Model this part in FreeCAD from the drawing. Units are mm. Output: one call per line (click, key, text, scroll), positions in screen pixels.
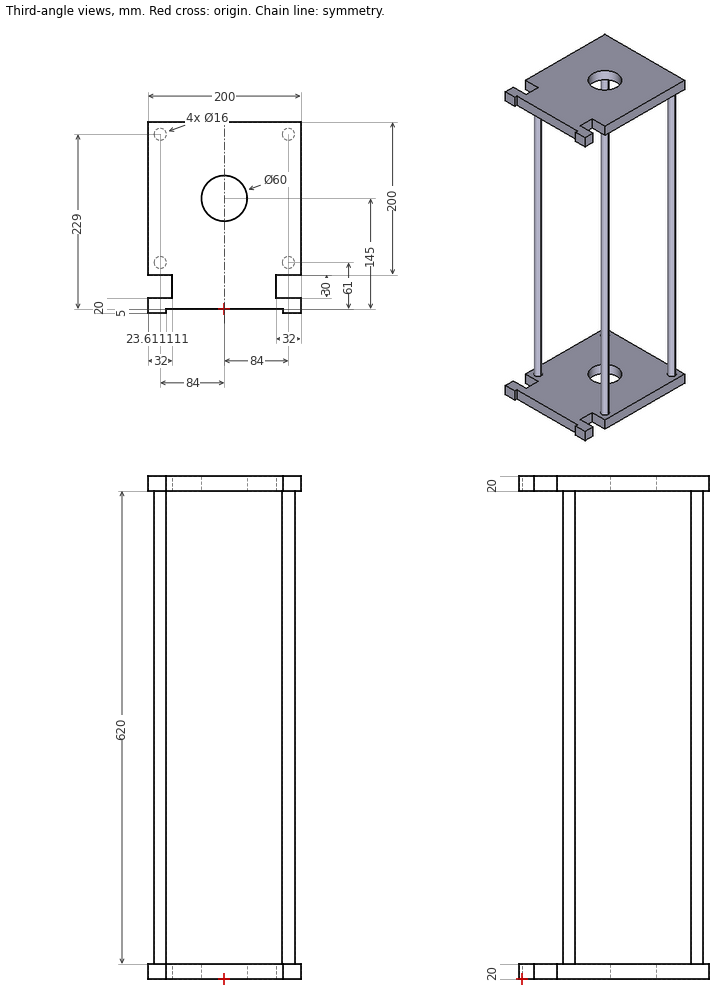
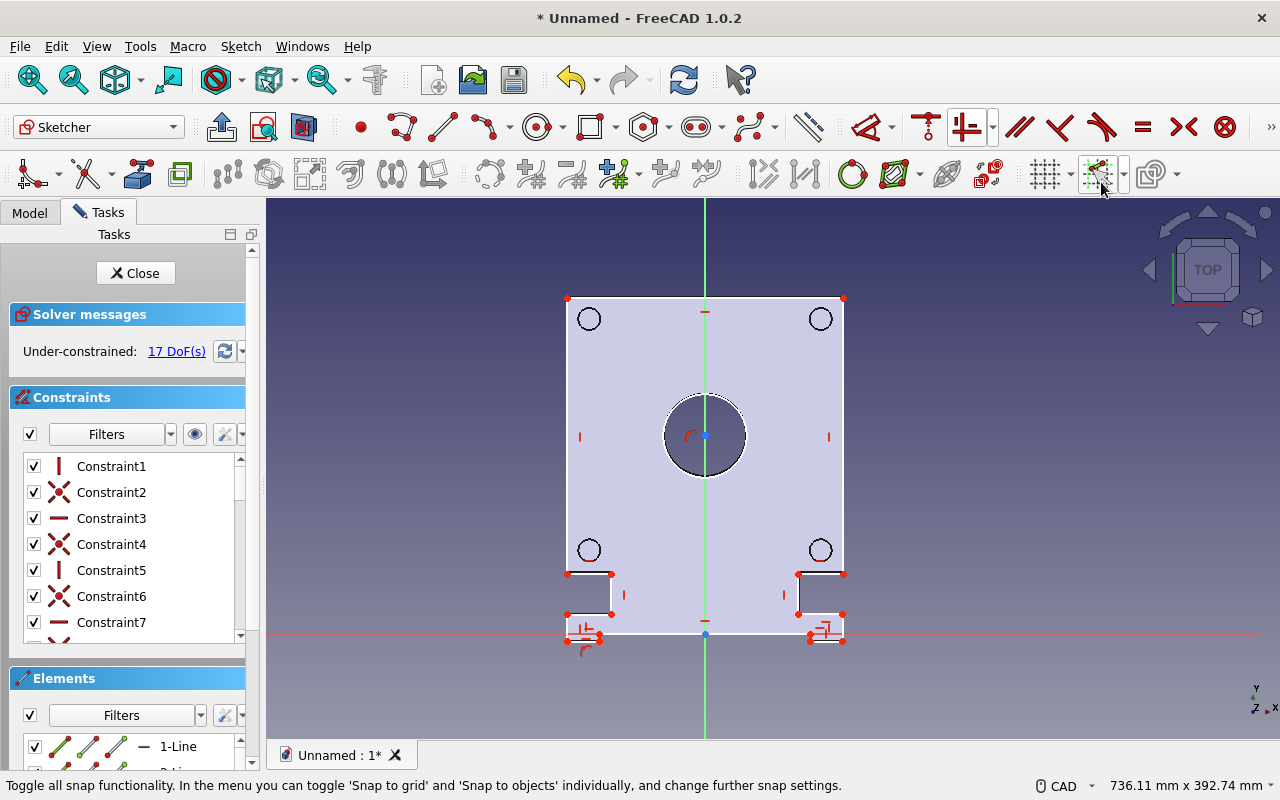
click(843, 574)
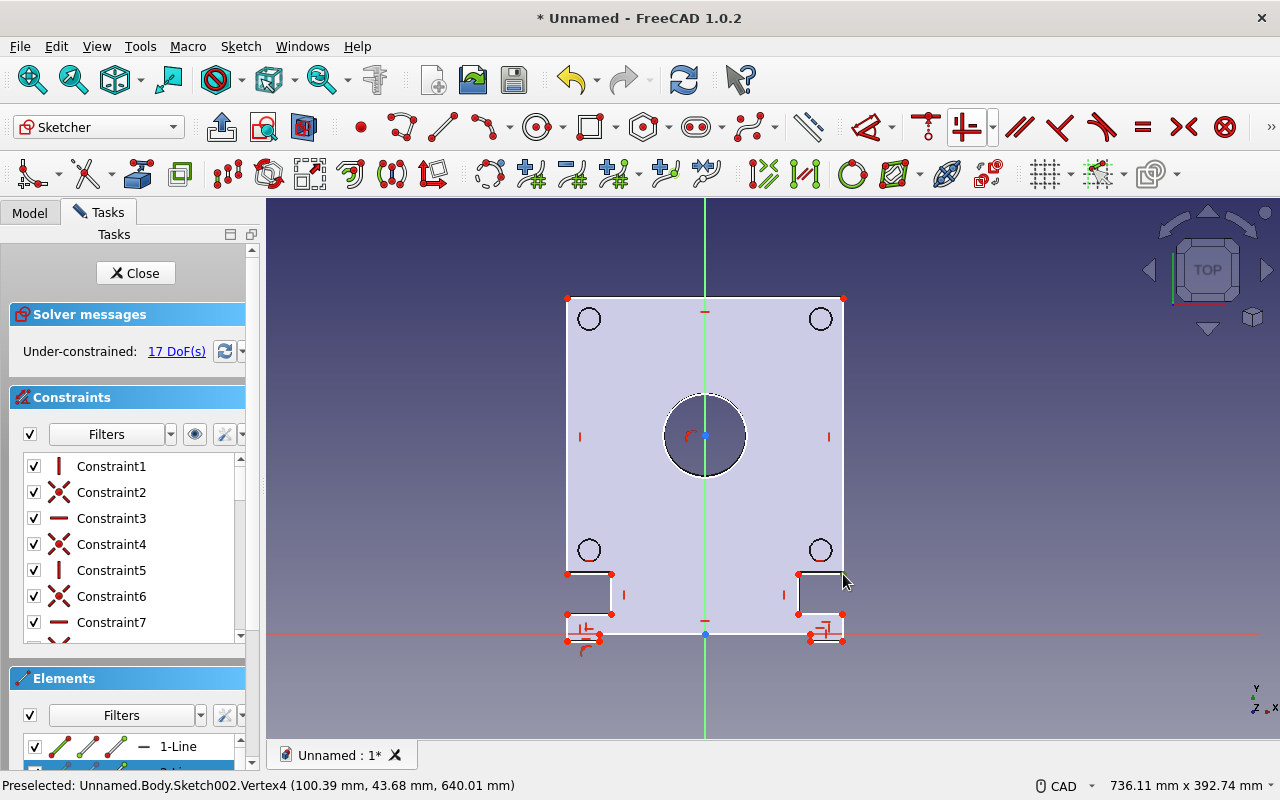
click(567, 574)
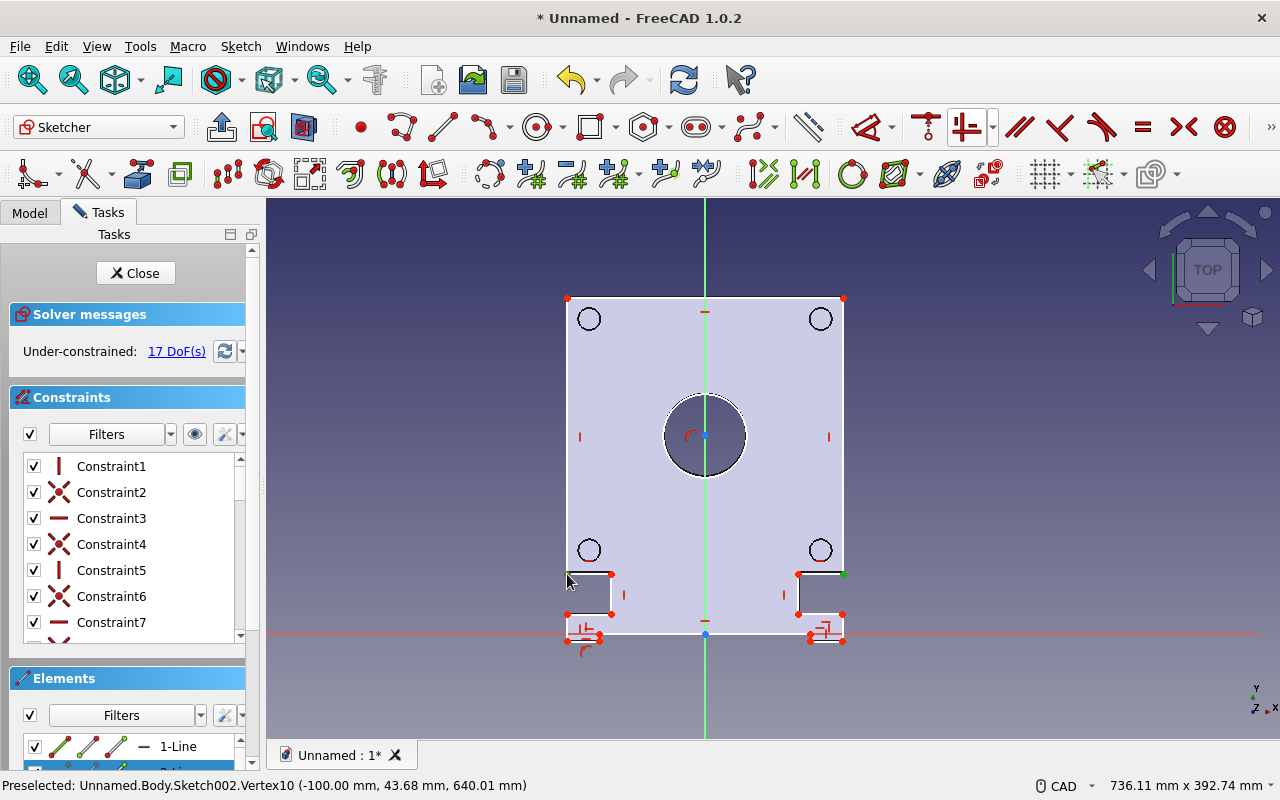
click(705, 676)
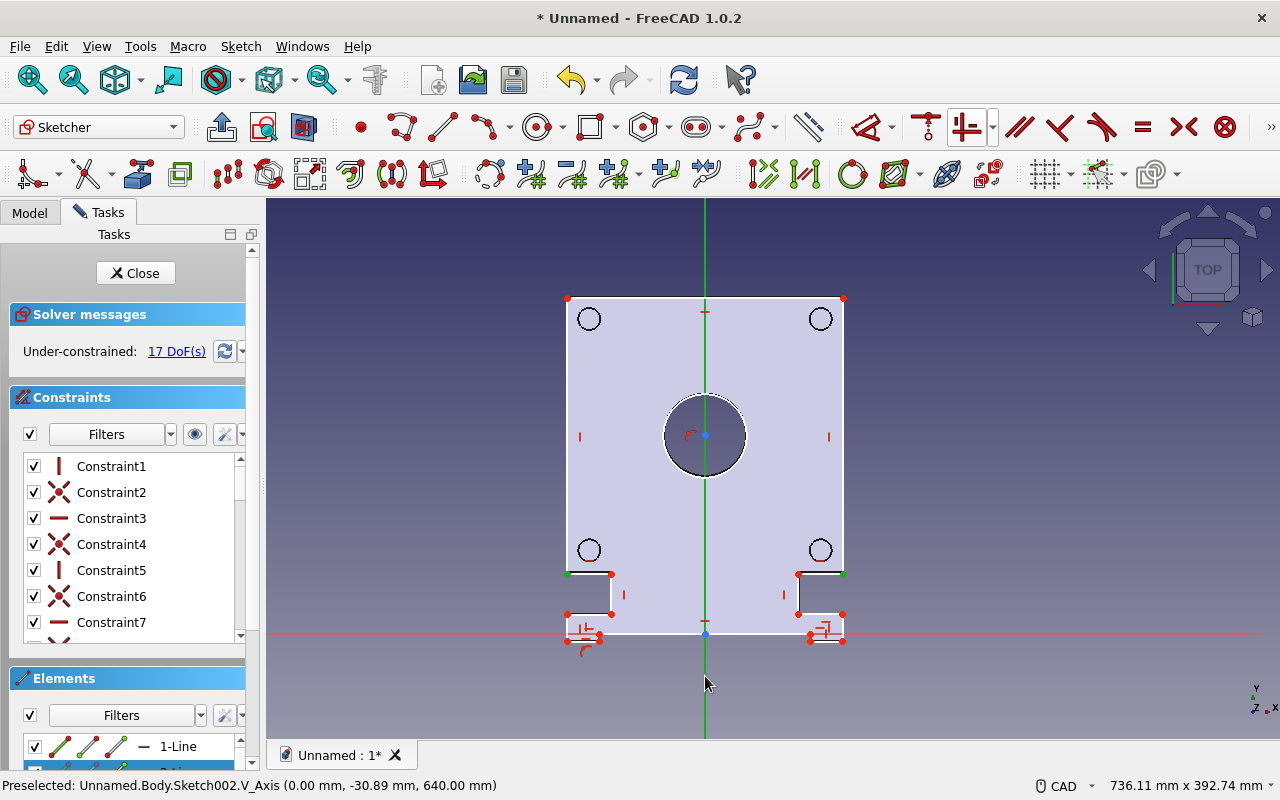
click(1184, 128)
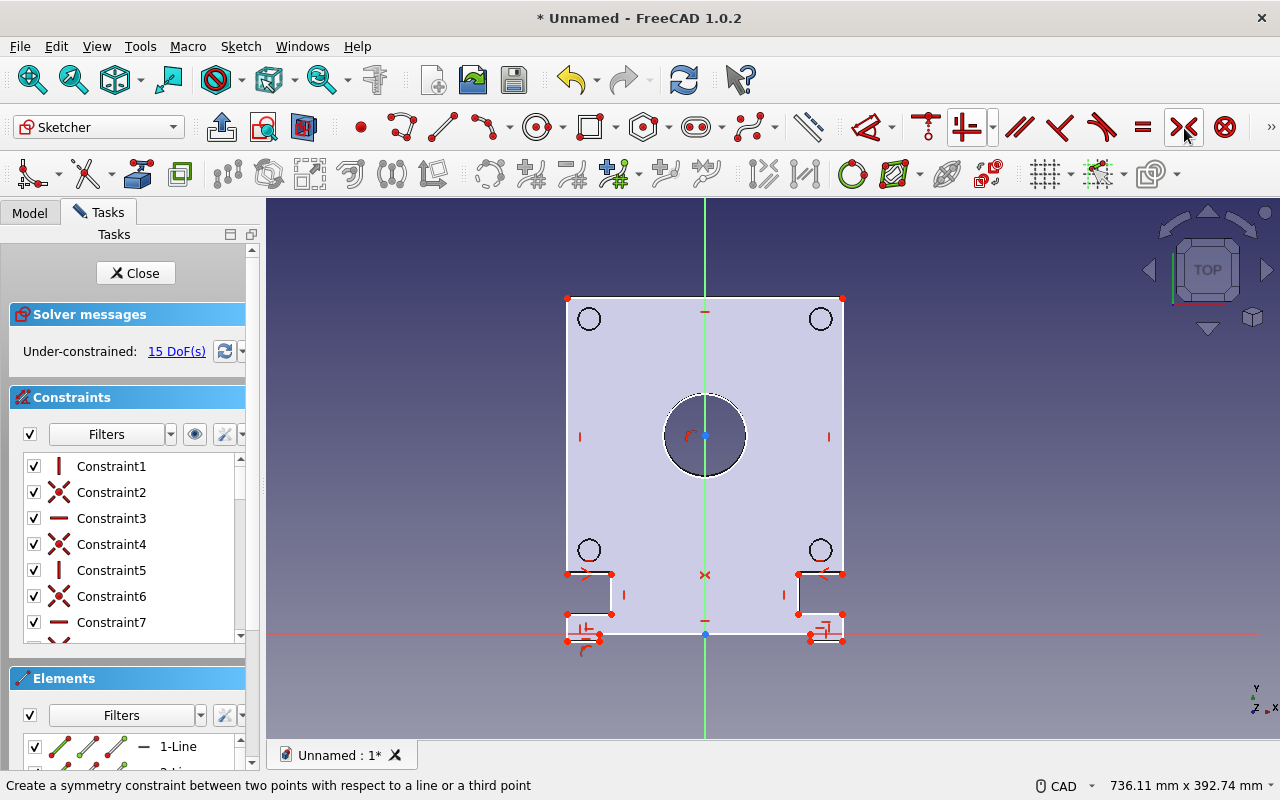
click(798, 614)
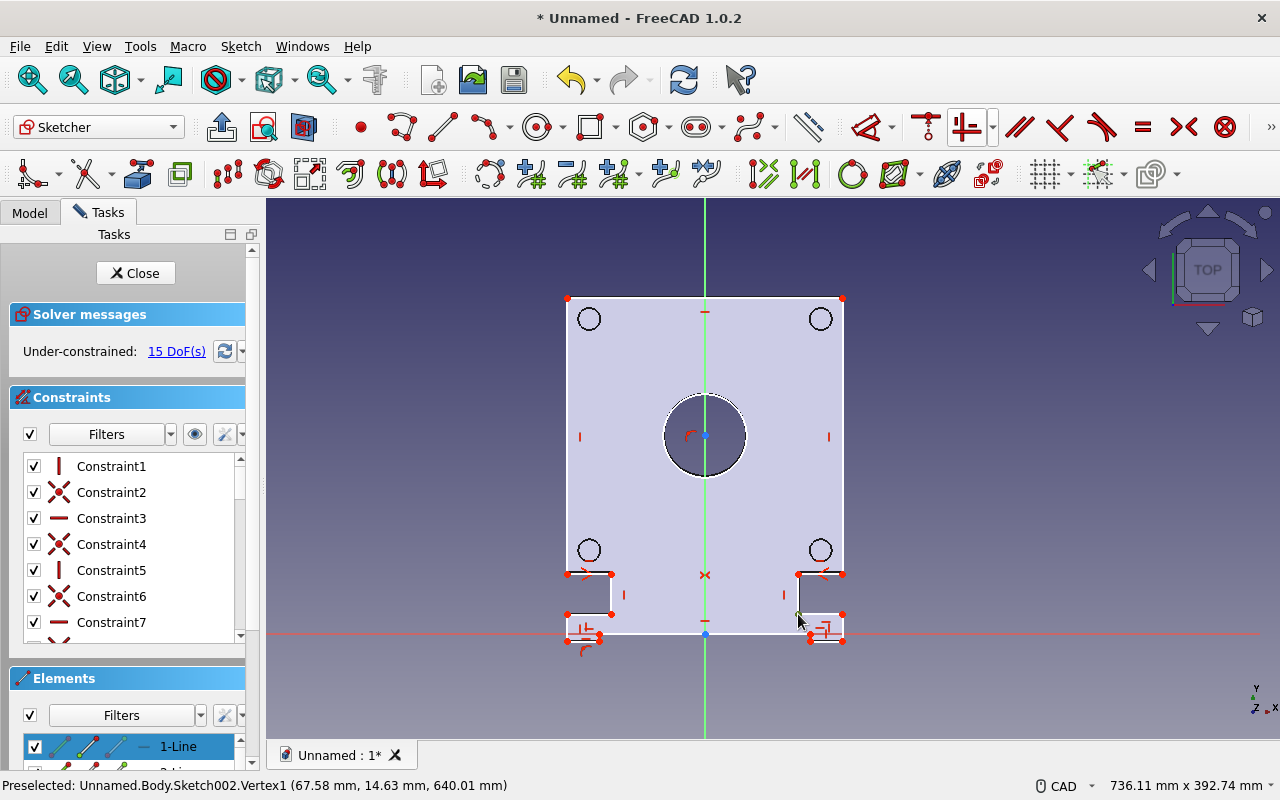
click(611, 615)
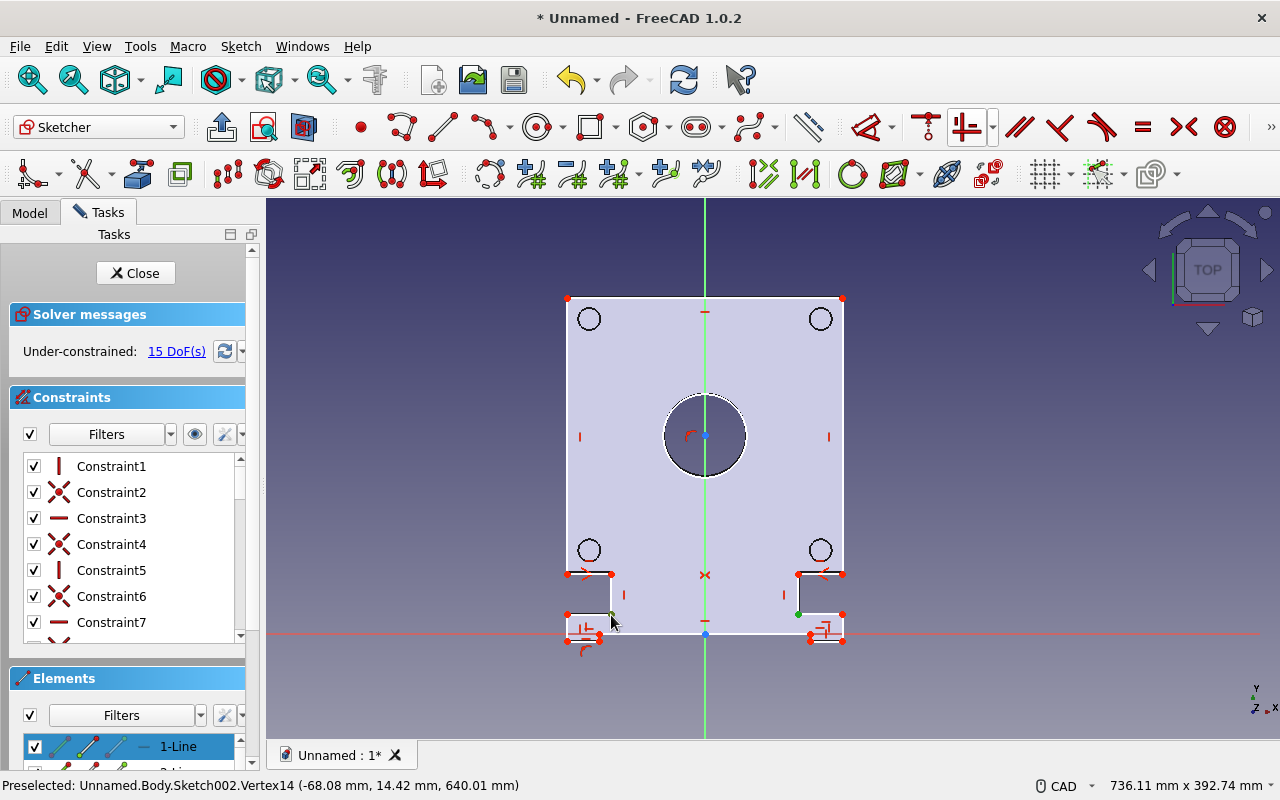
click(705, 676)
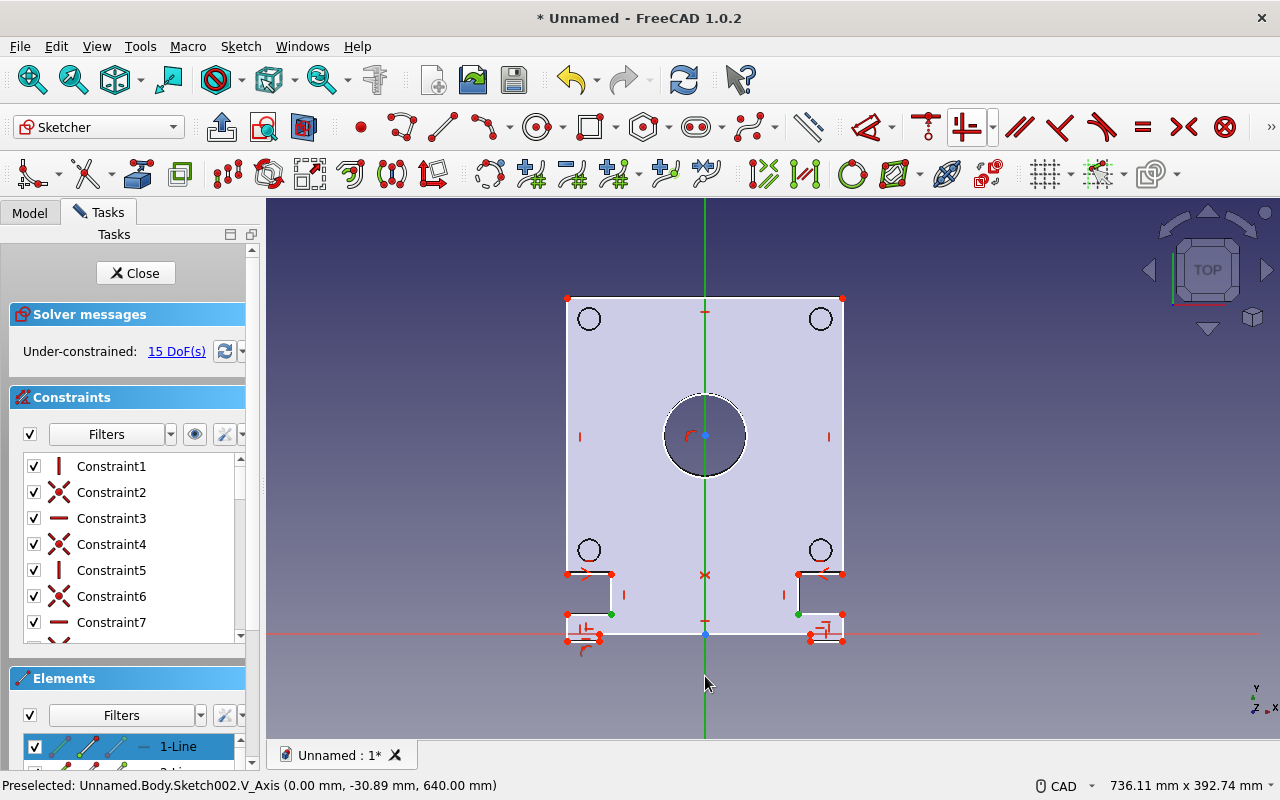
click(1184, 128)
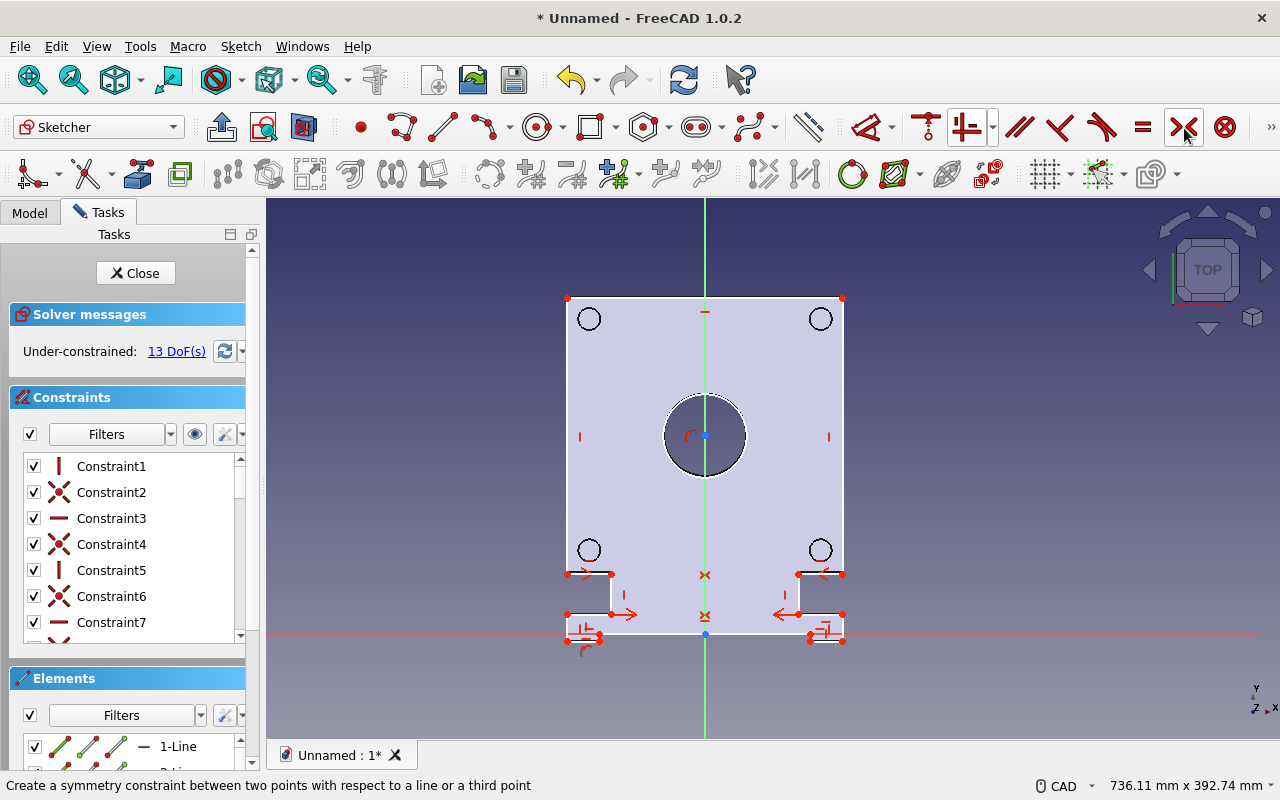
scroll(600, 642, up, 3)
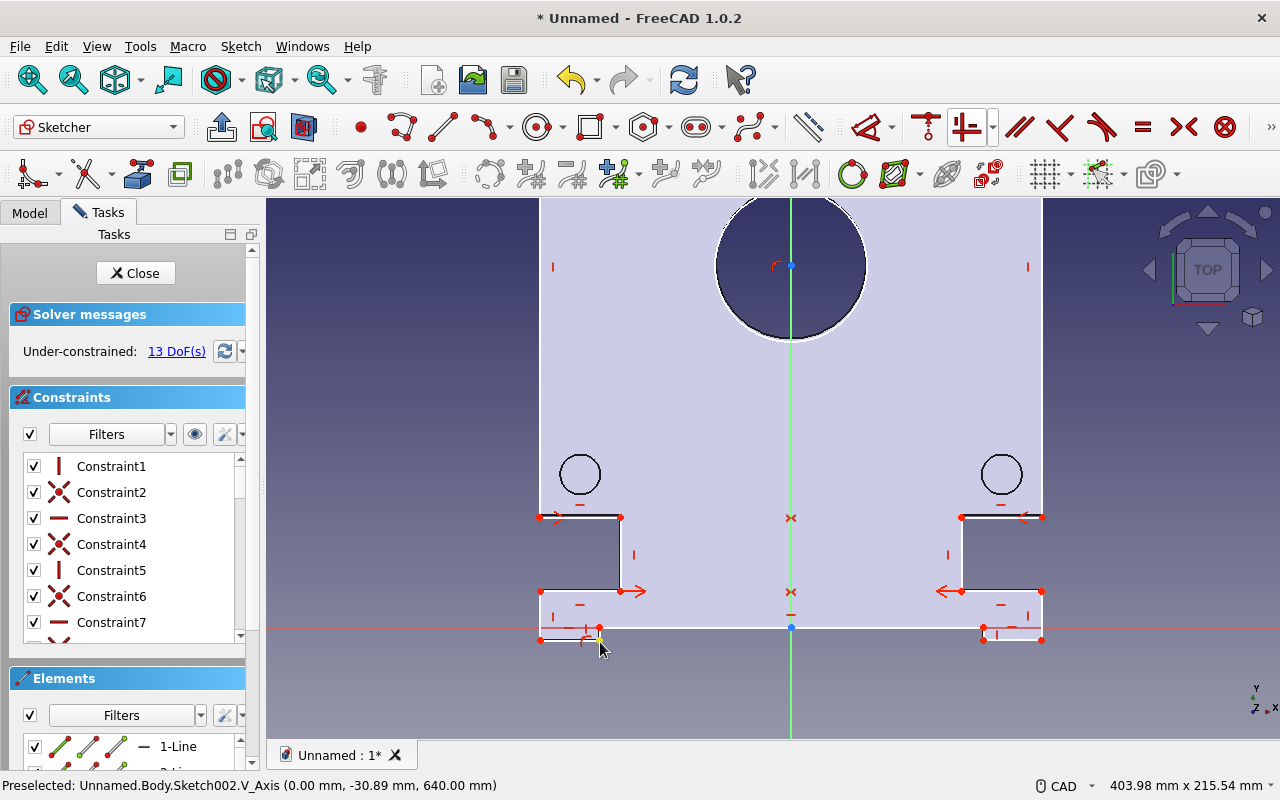
click(600, 641)